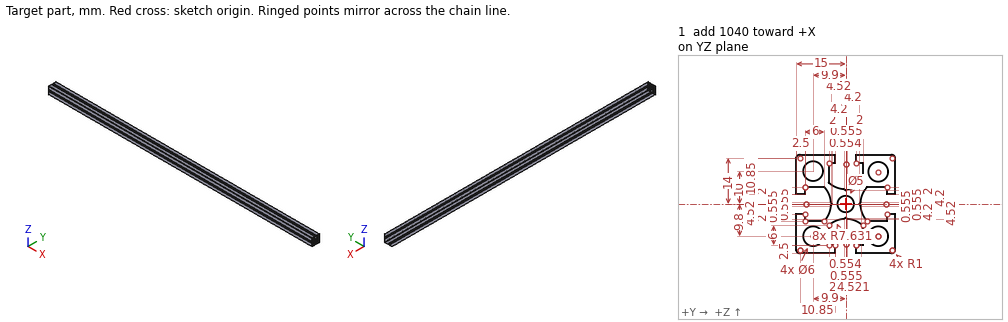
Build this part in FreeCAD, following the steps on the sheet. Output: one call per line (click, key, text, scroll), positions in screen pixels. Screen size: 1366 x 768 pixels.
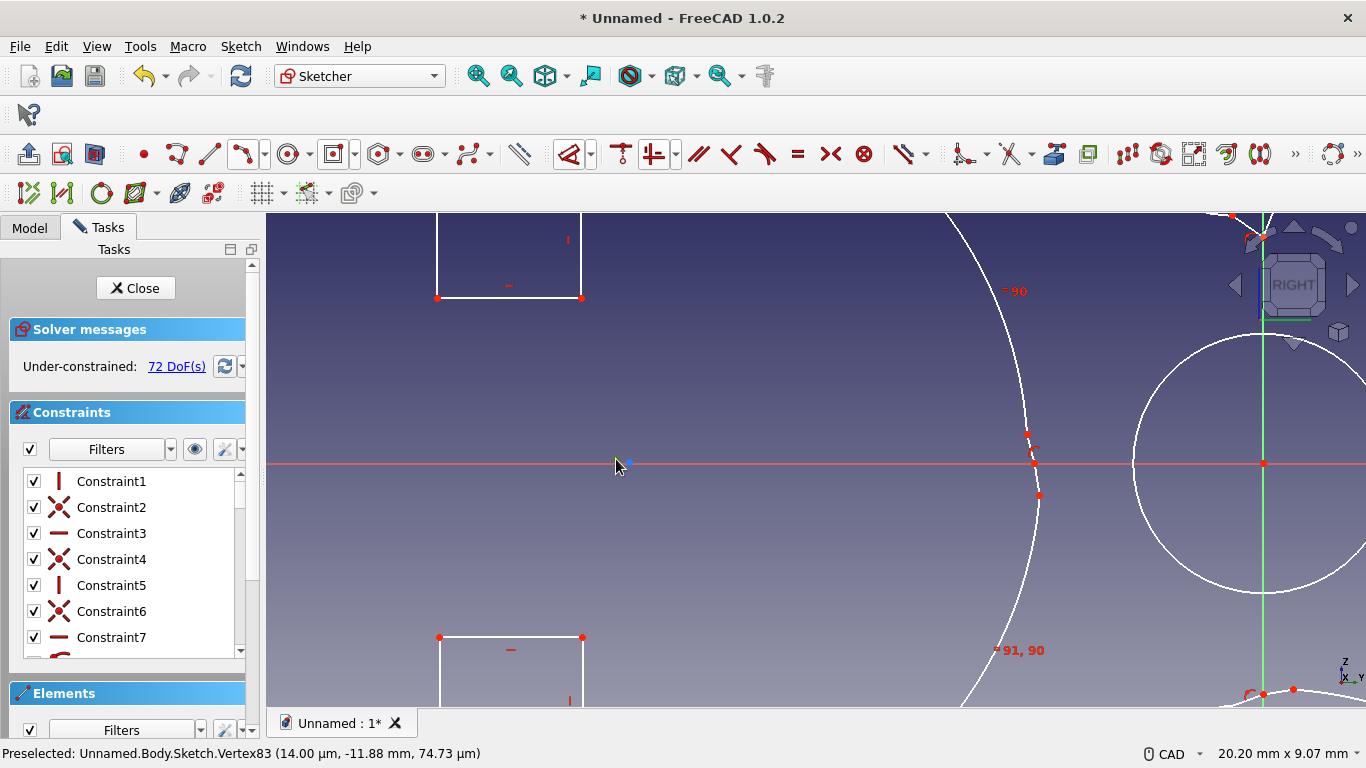
click(629, 462)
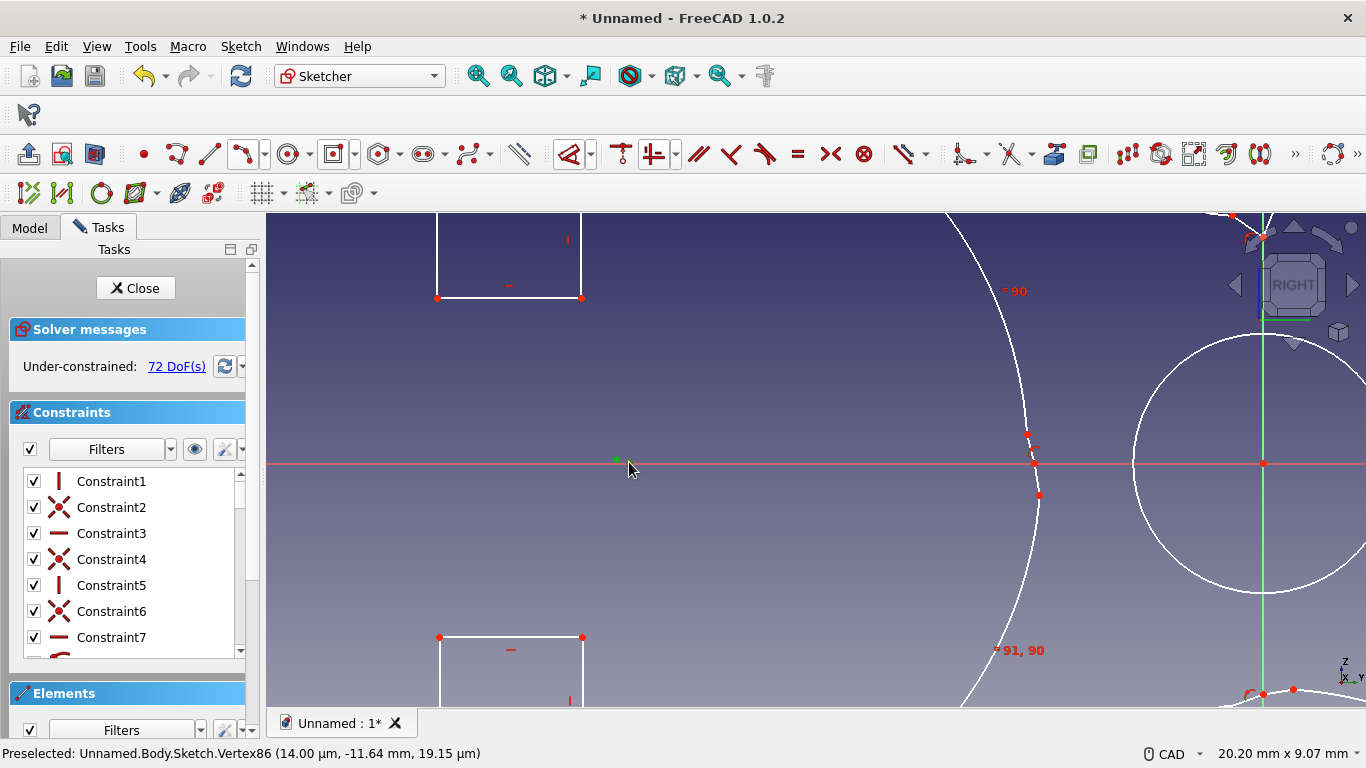
click(359, 464)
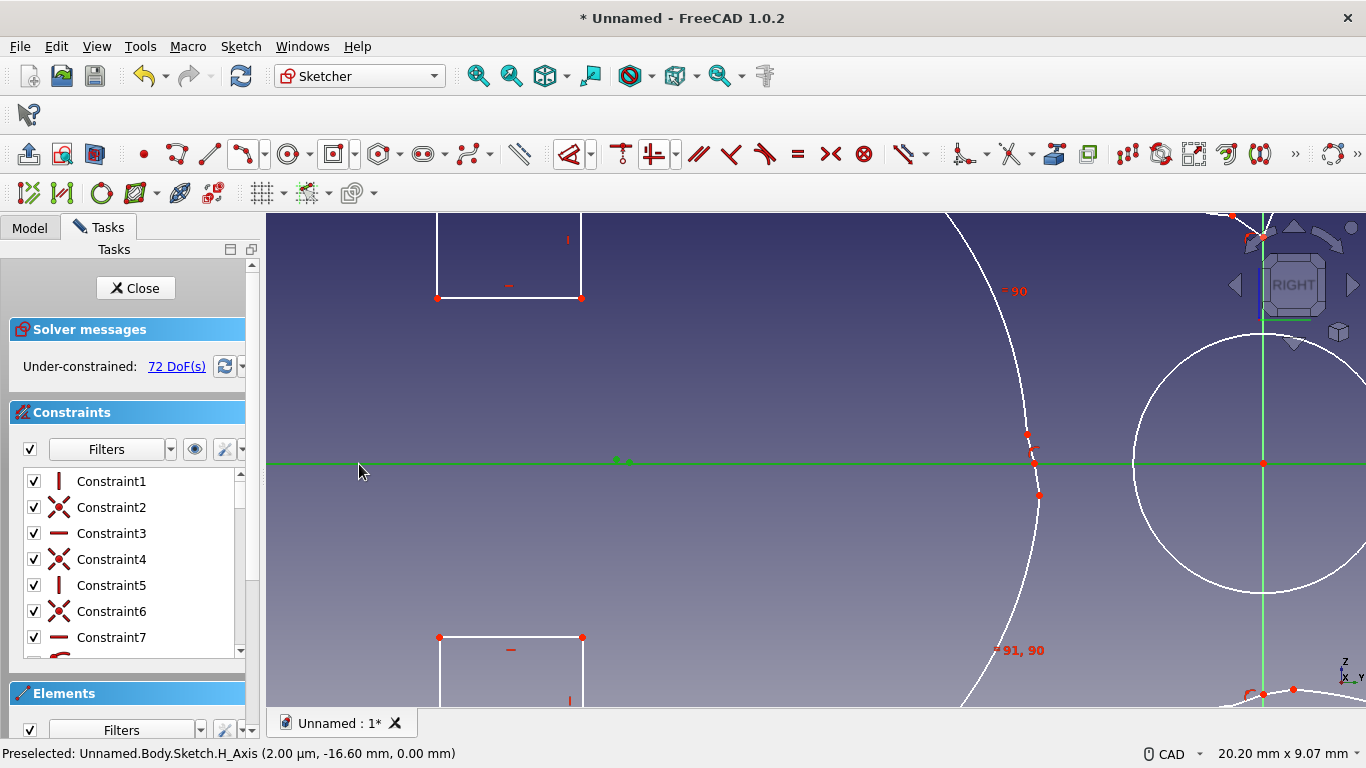
key(s)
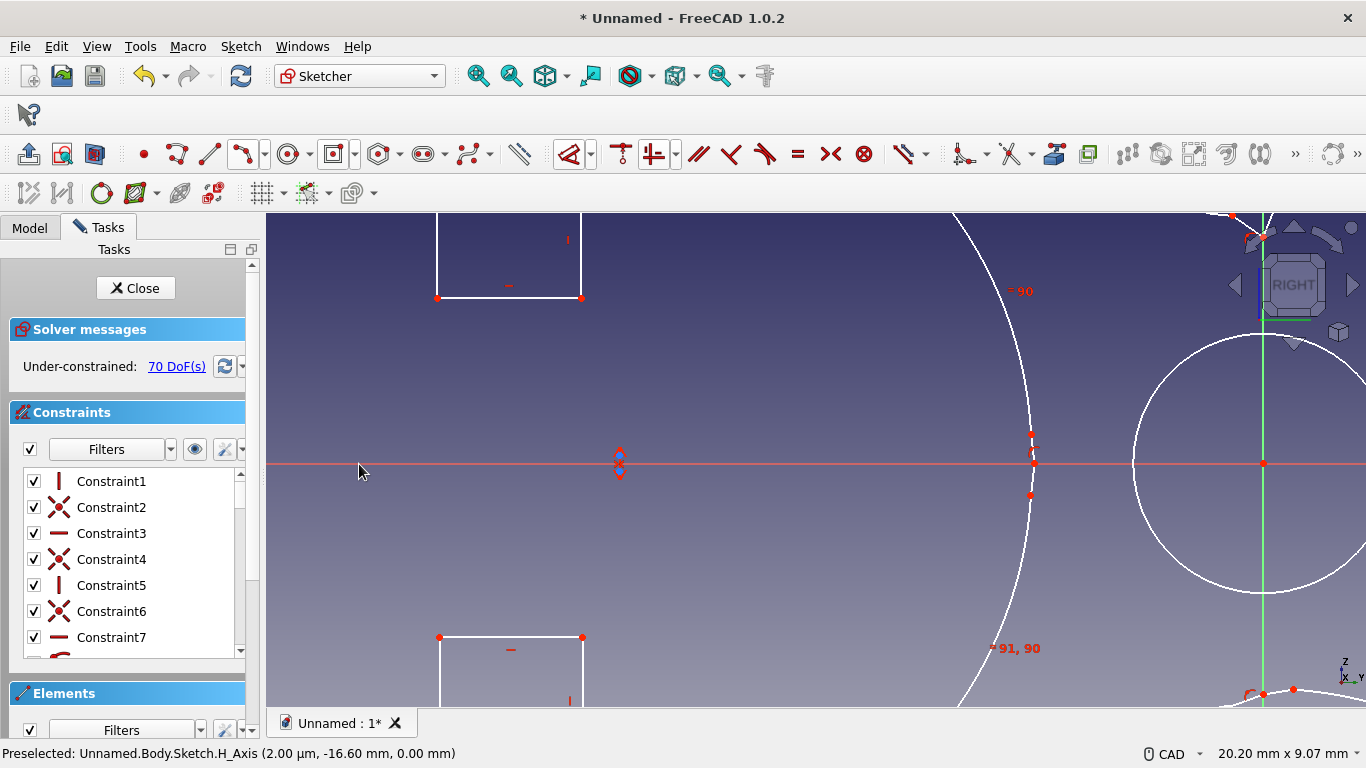
scroll(617, 459, down, 8)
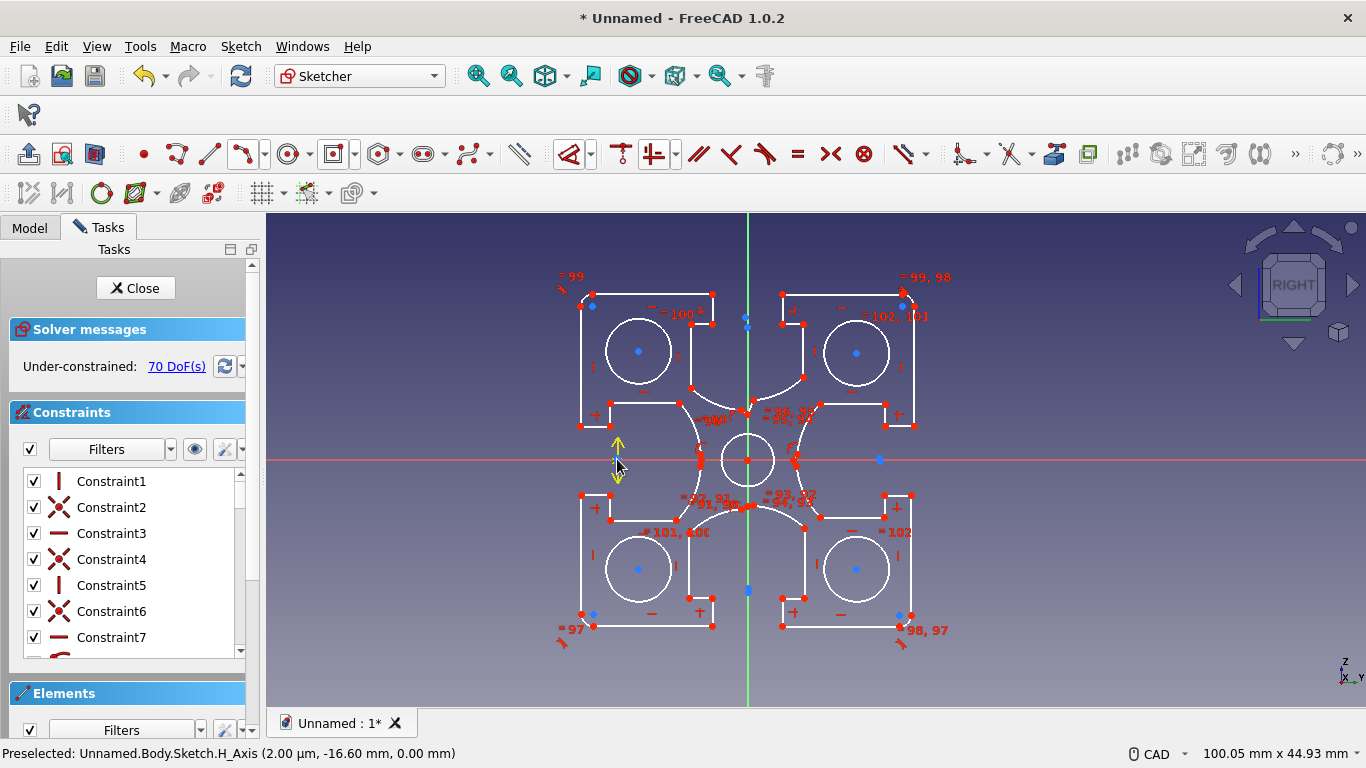
click(593, 614)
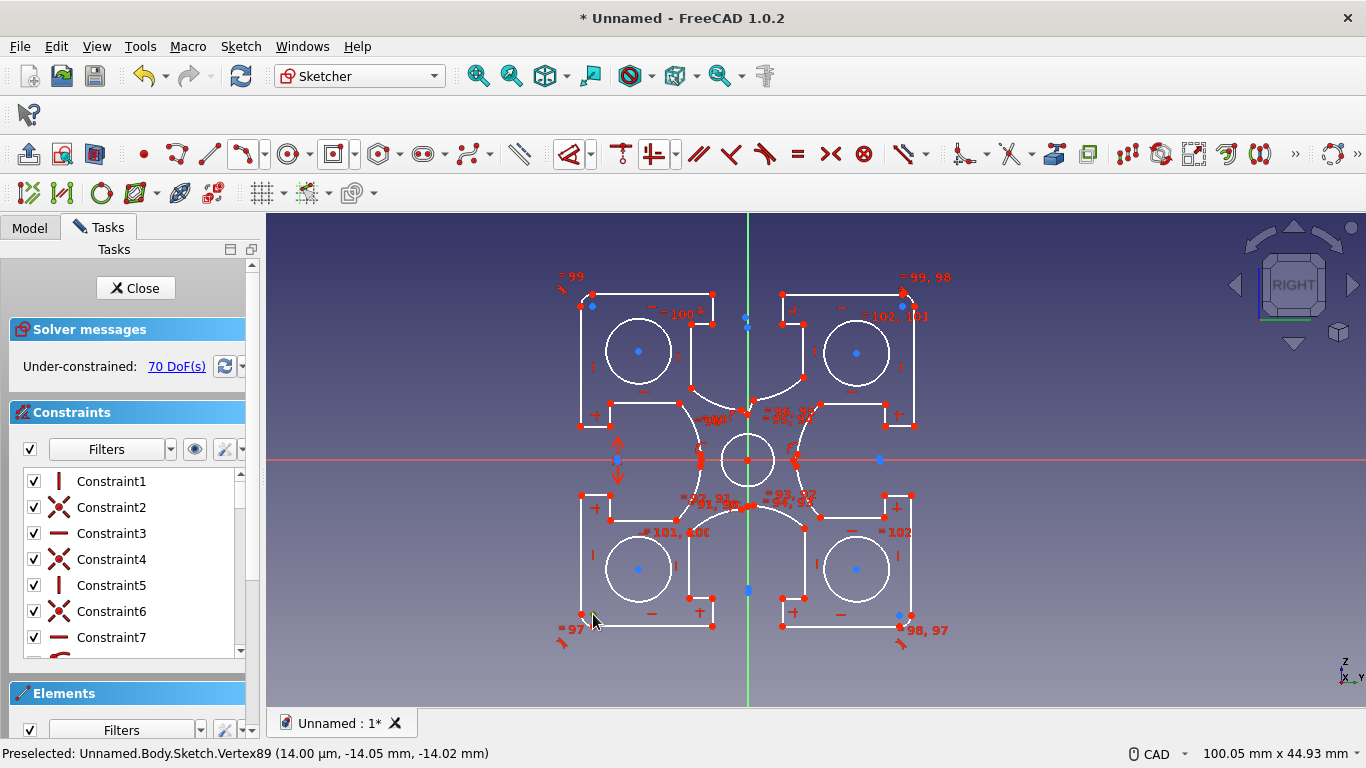
click(900, 615)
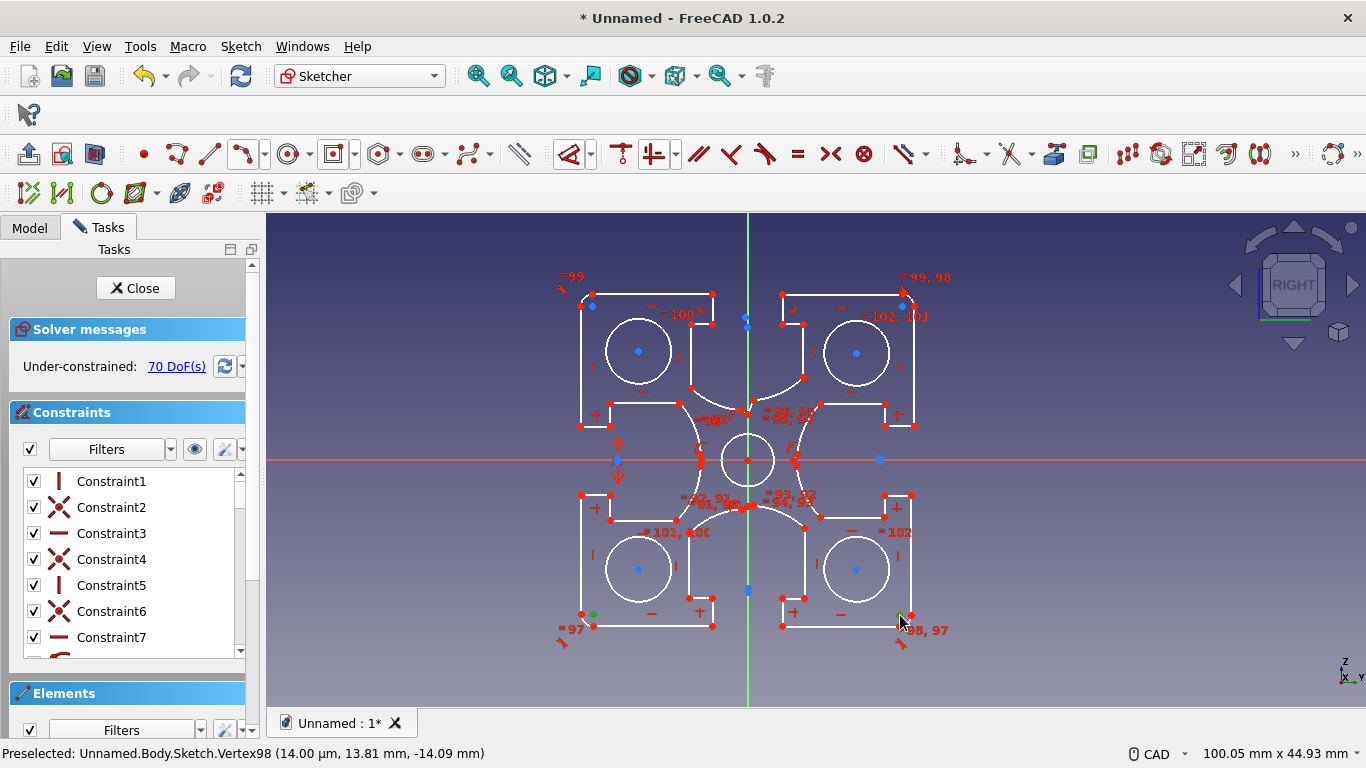
click(748, 648)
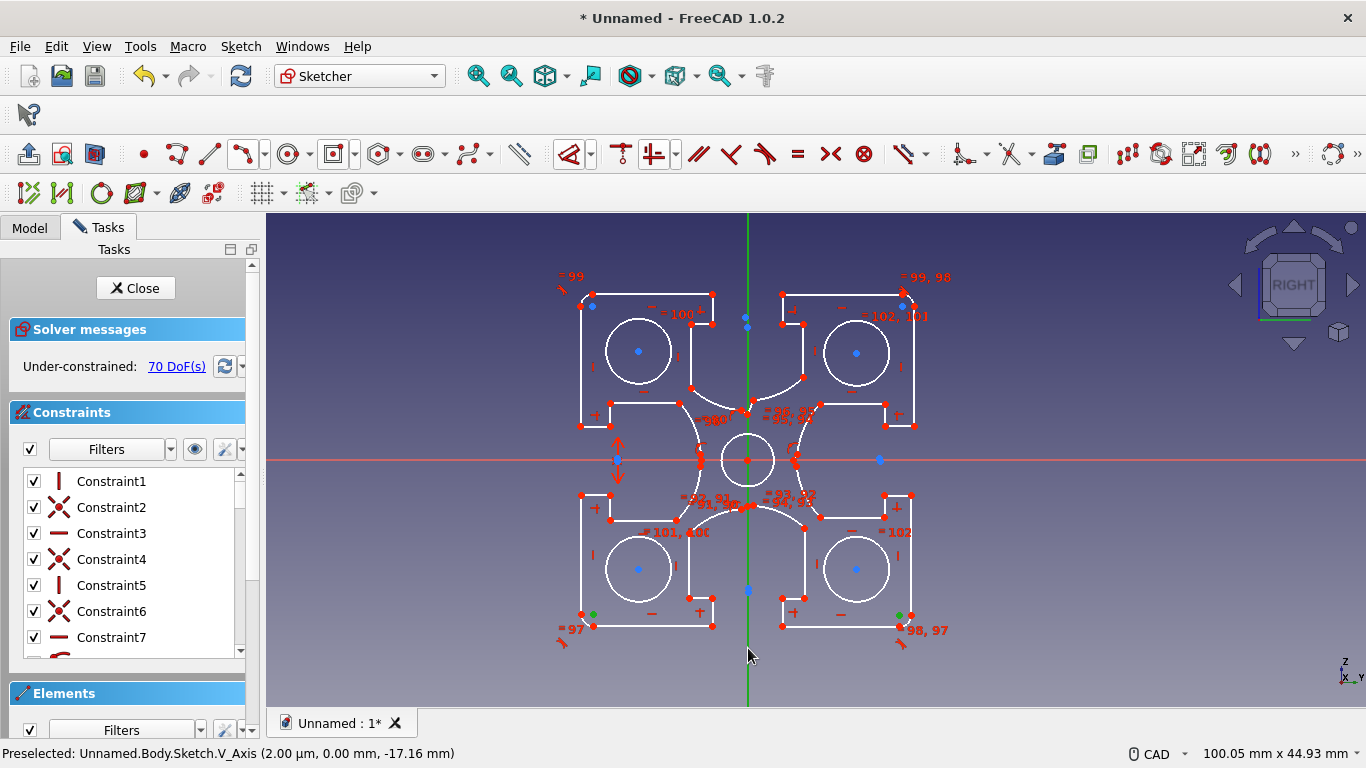
key(s)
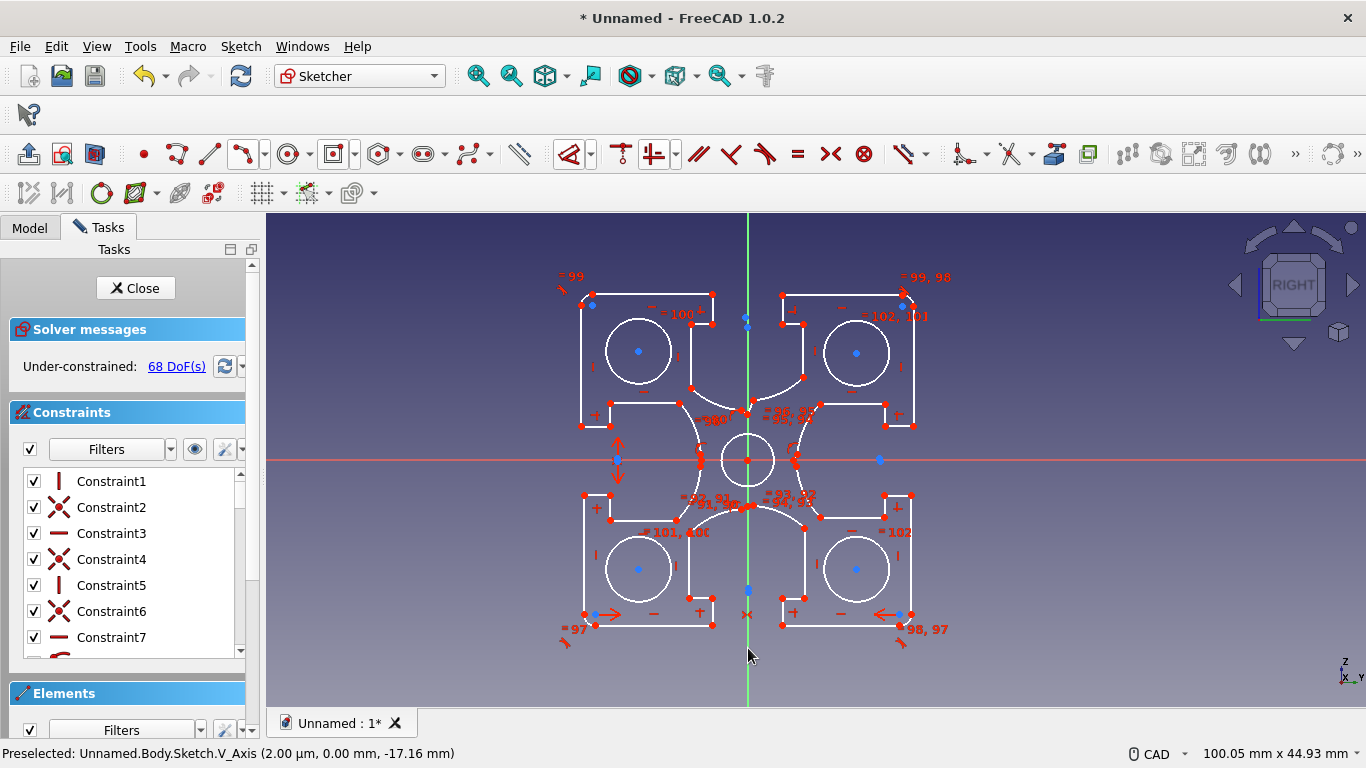
scroll(880, 459, up, 8)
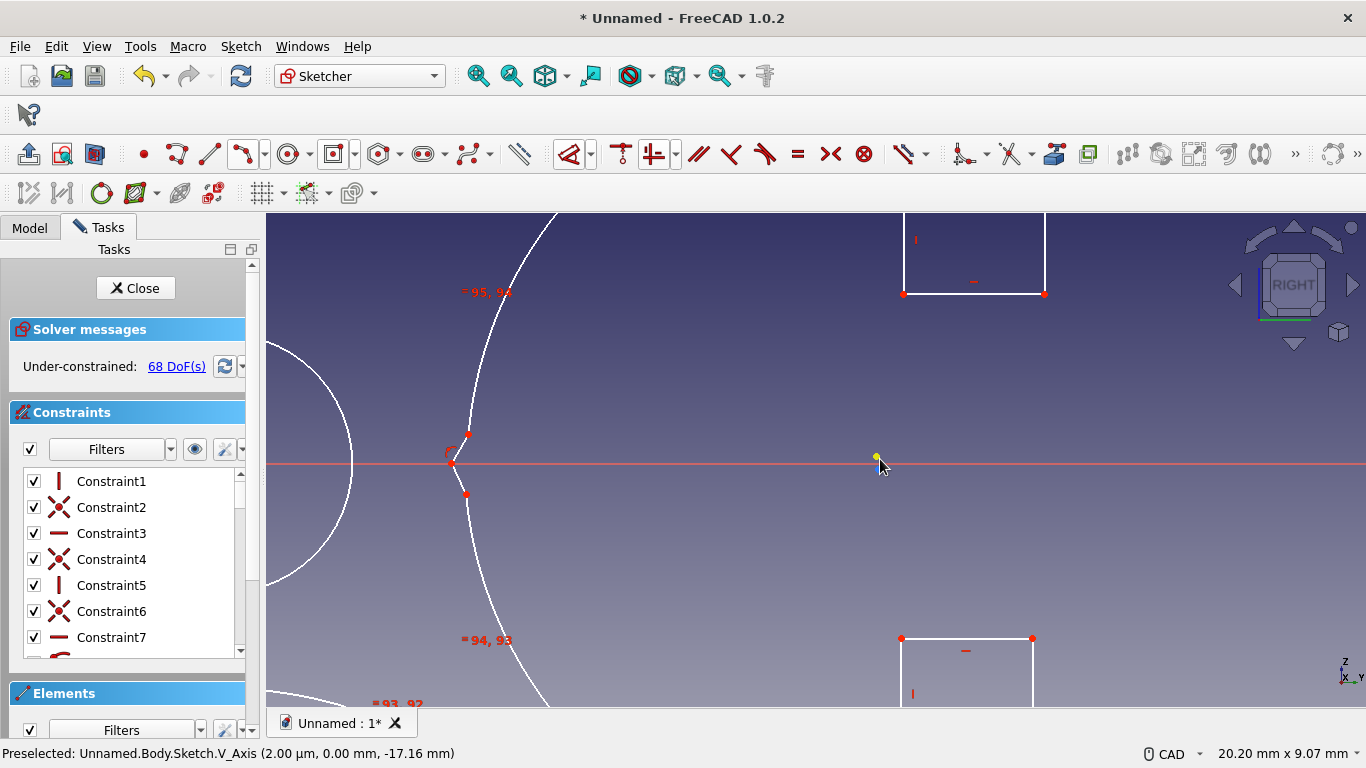
click(876, 457)